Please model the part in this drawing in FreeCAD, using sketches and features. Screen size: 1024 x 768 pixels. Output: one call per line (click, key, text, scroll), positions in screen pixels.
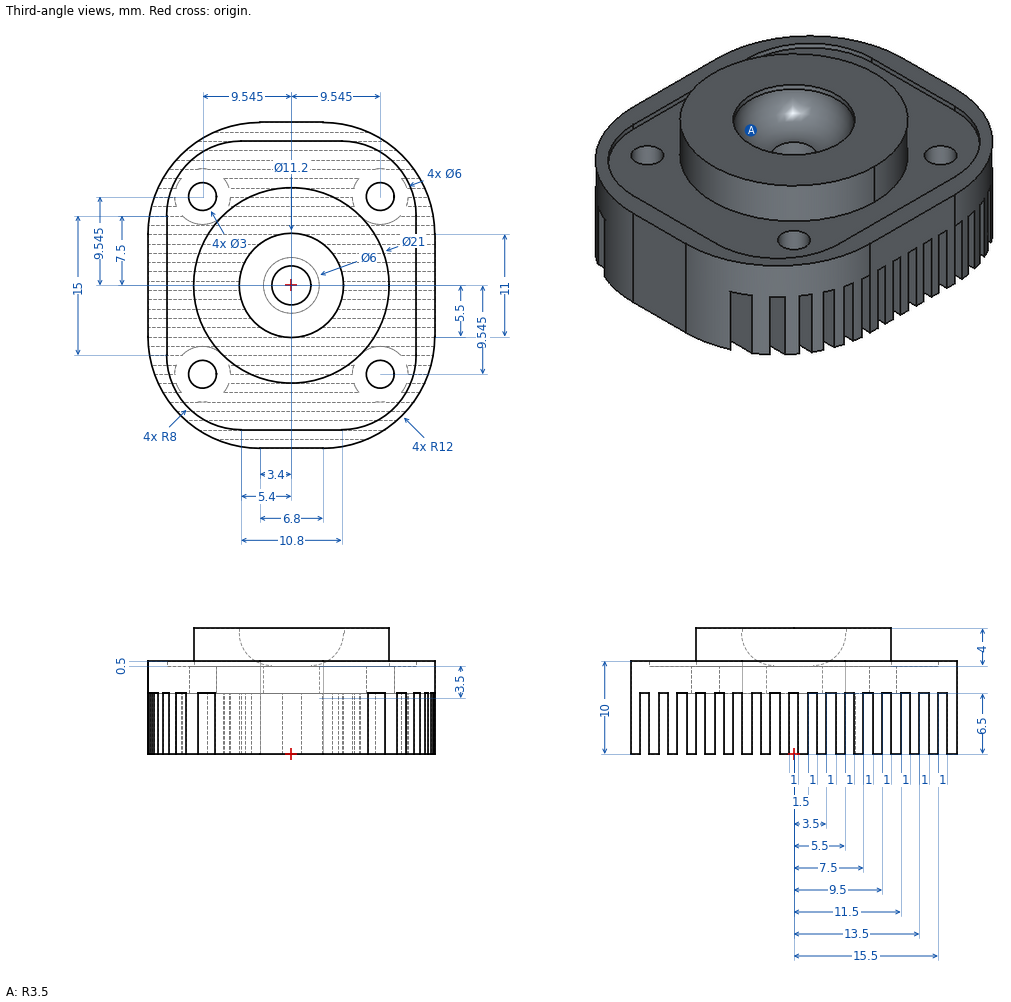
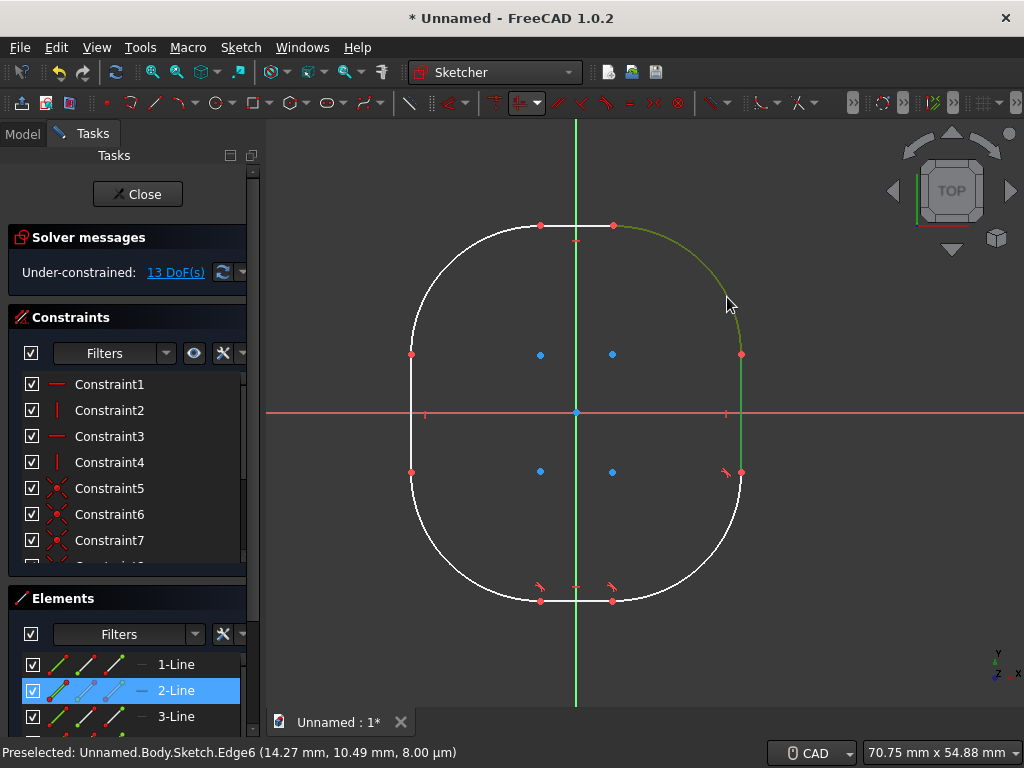
click(606, 104)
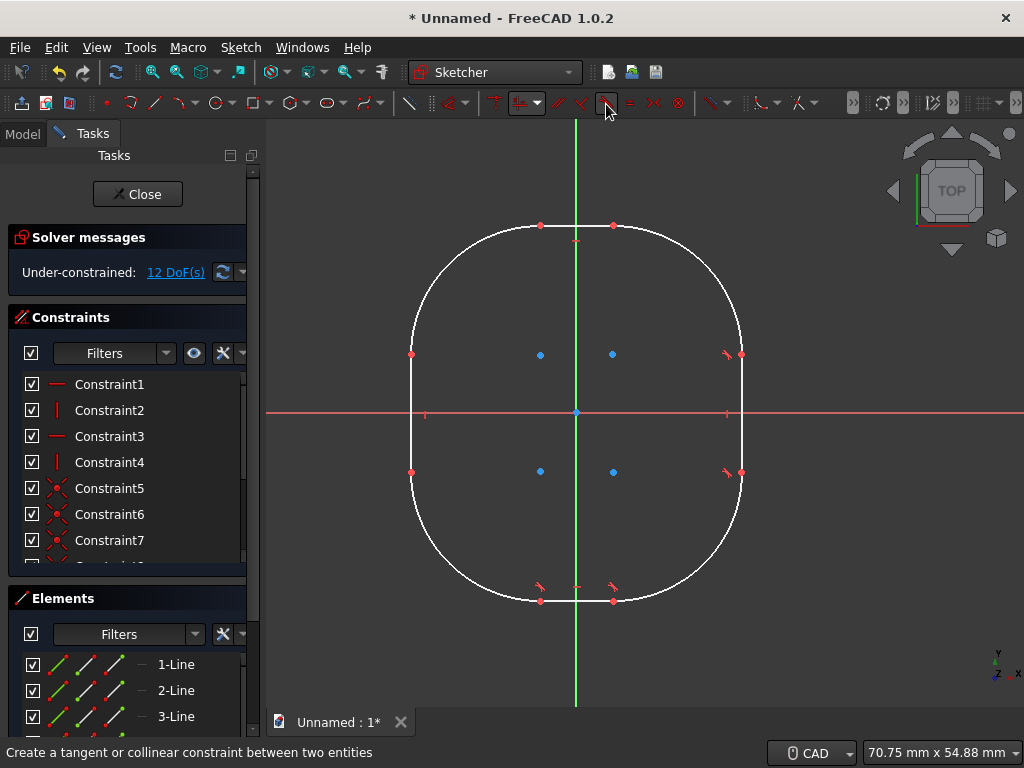
click(591, 226)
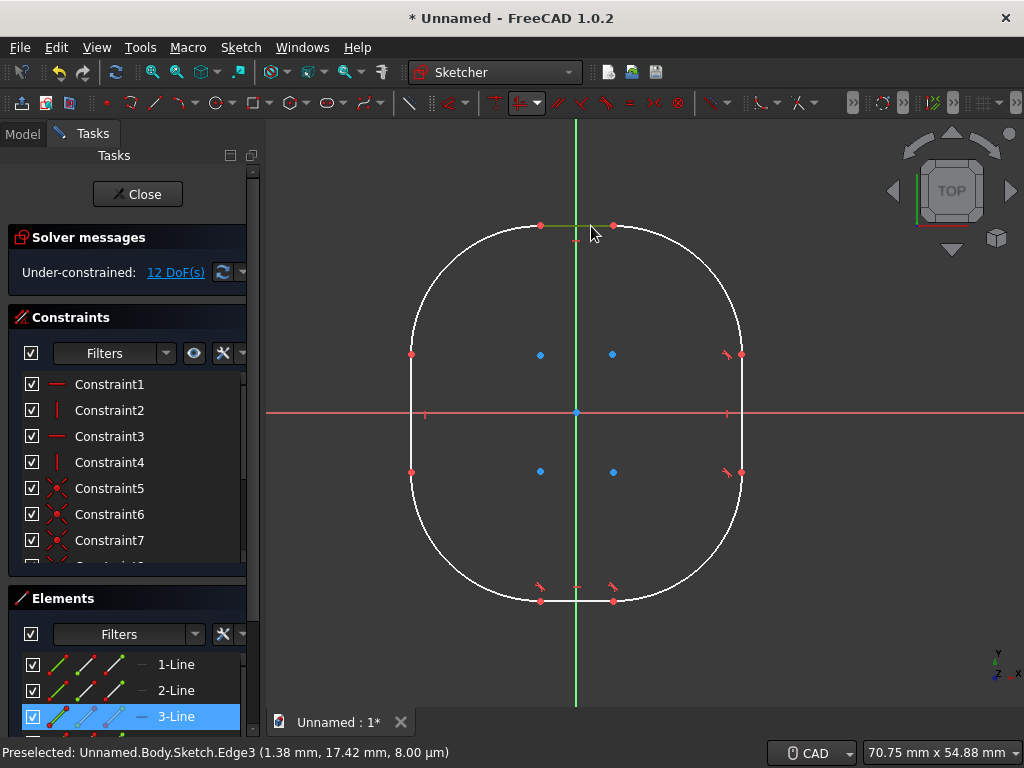
click(728, 296)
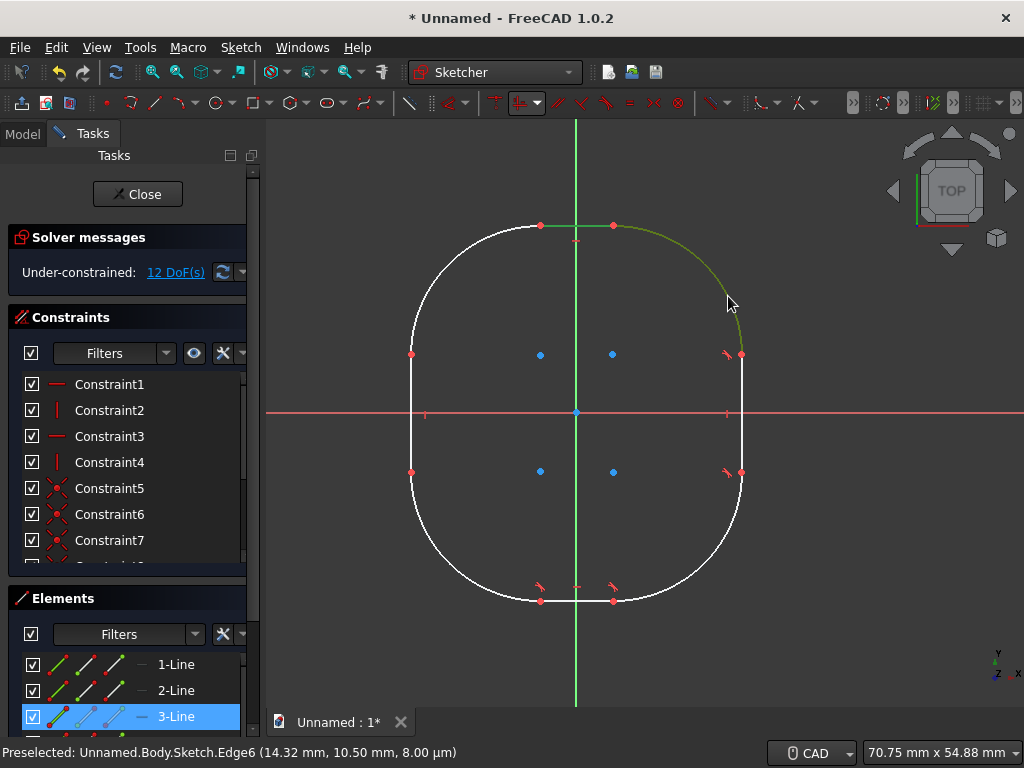
click(606, 104)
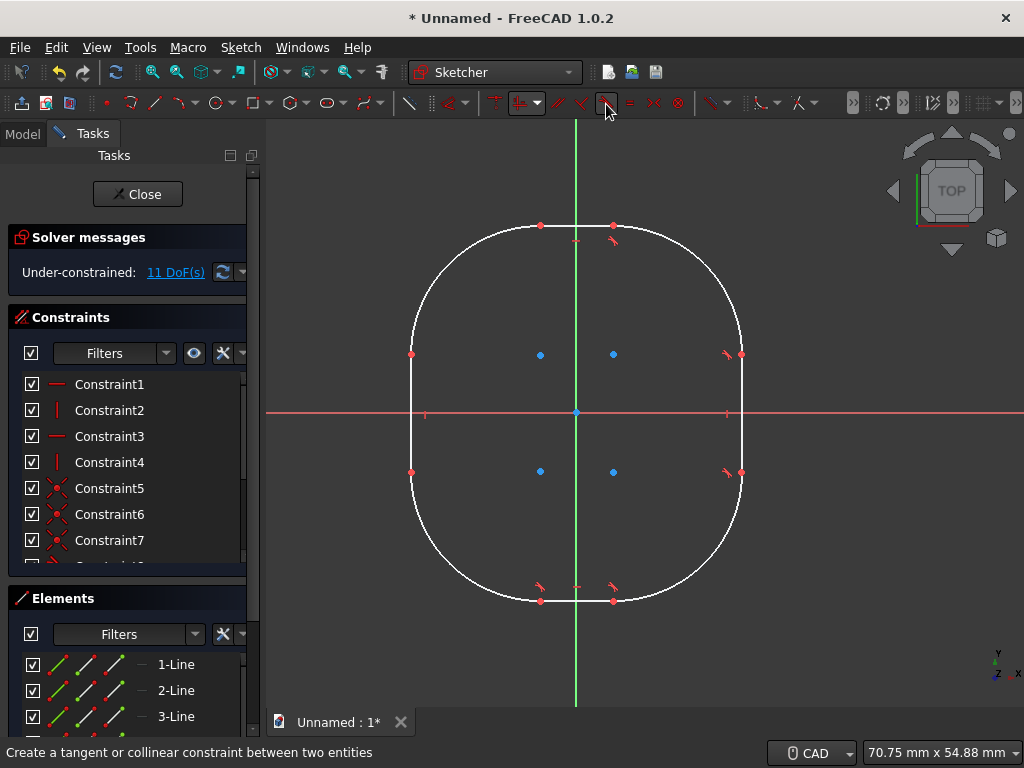
click(591, 226)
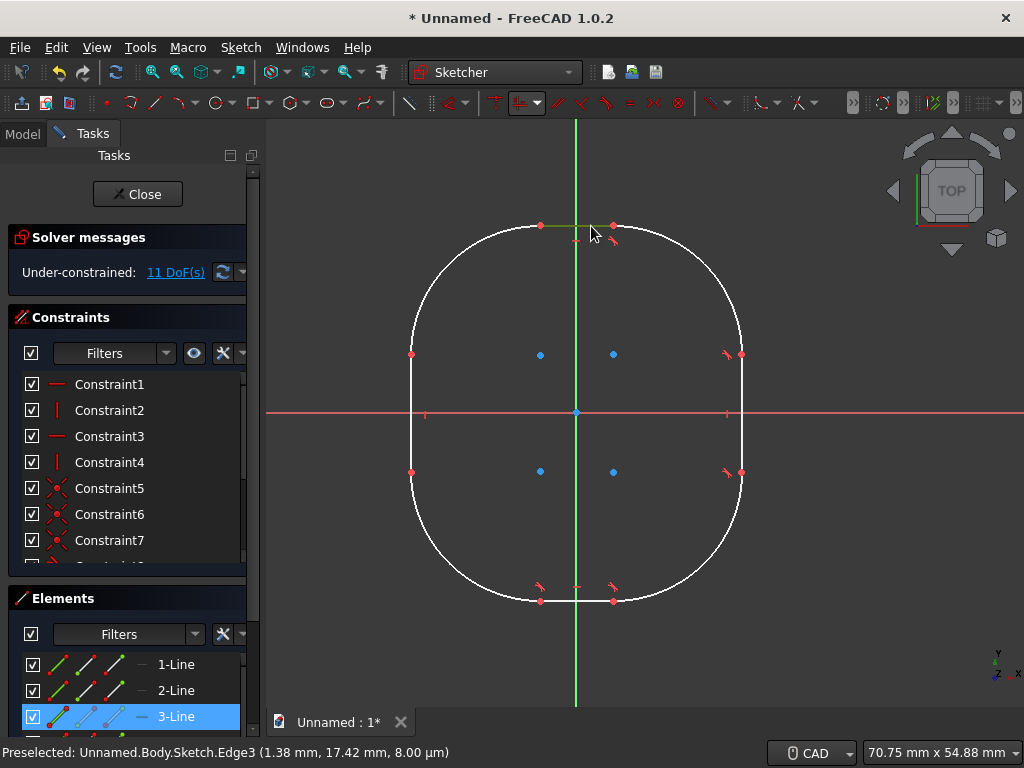
click(482, 240)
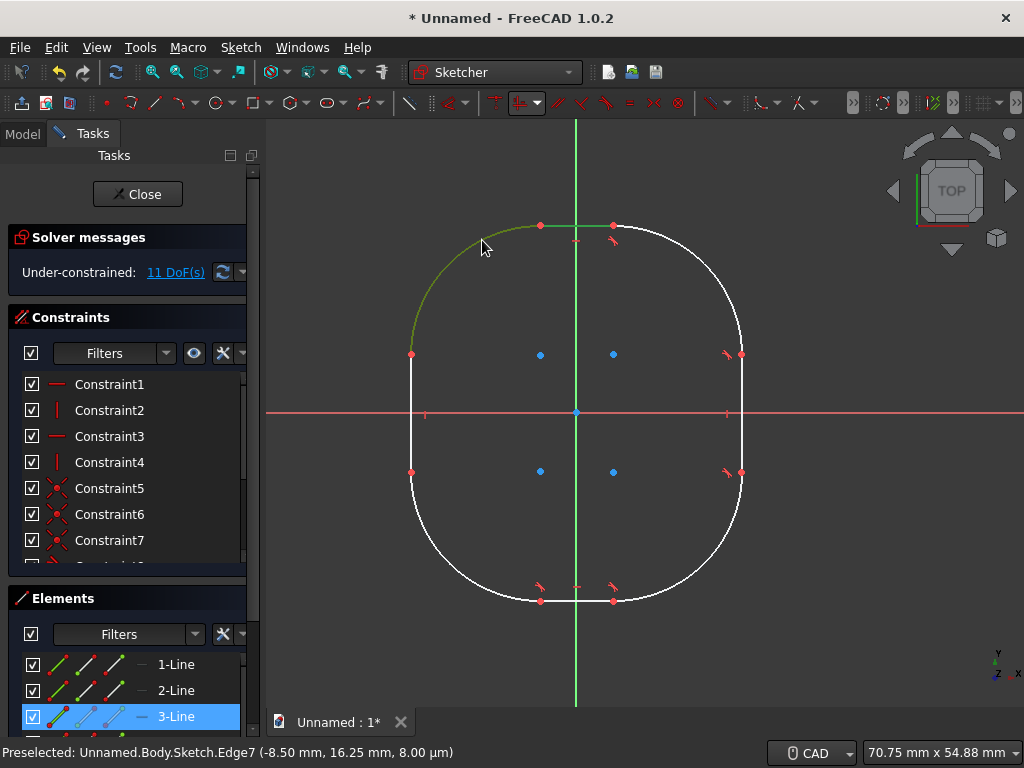
key(t)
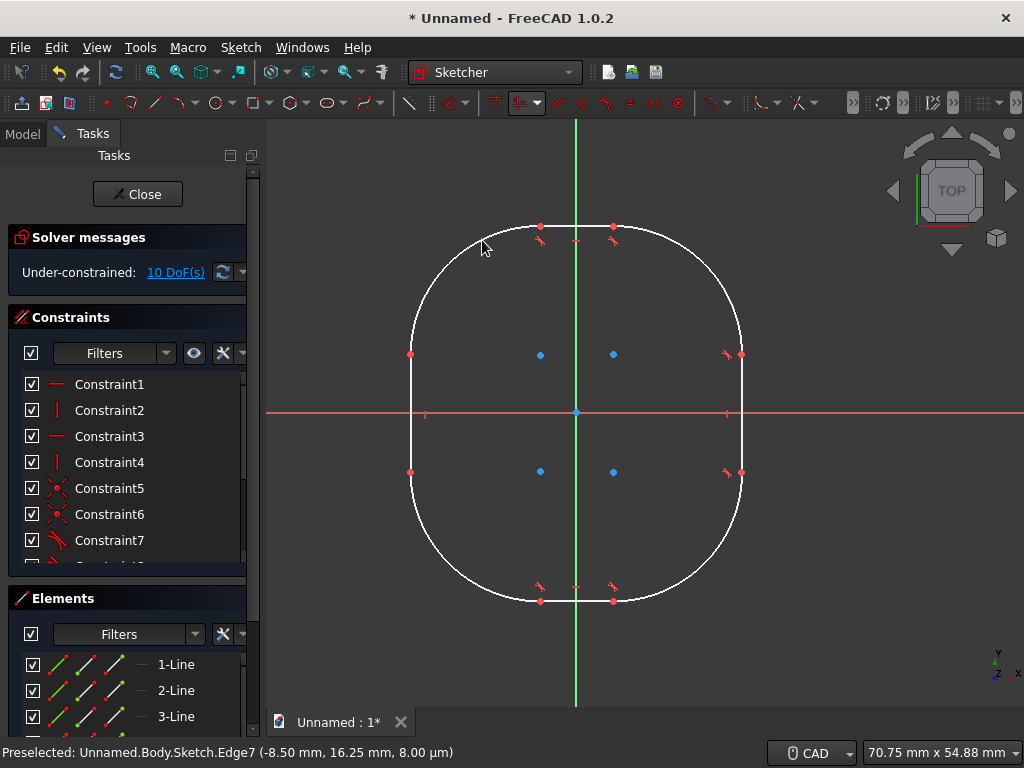
click(411, 390)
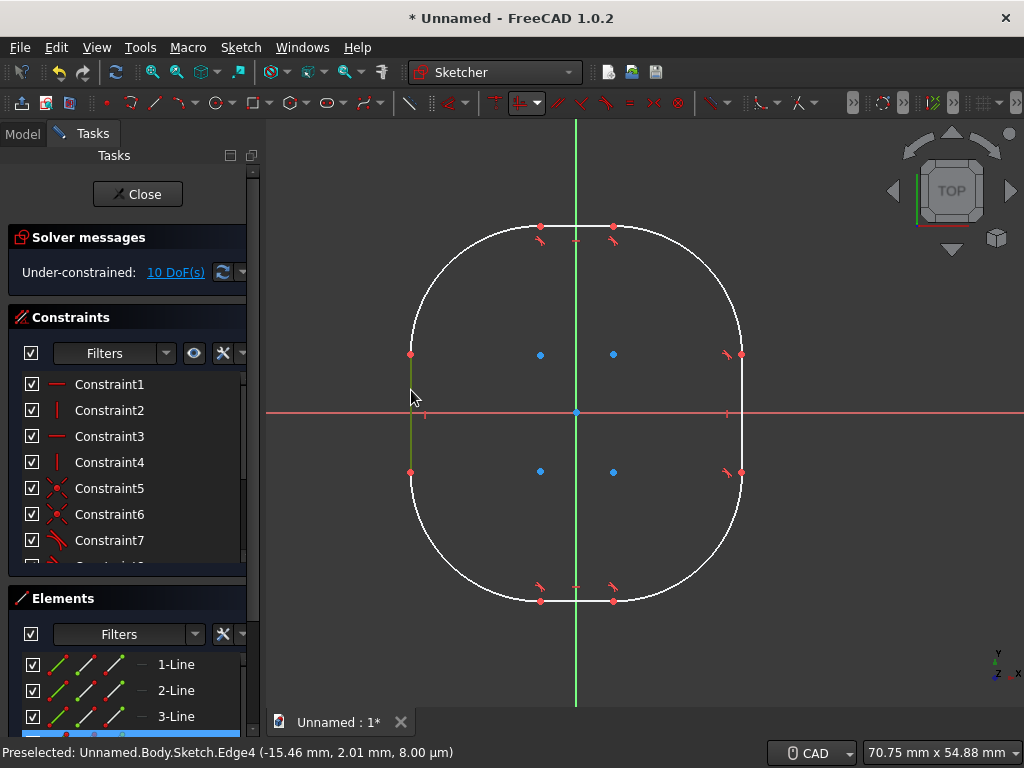
click(482, 240)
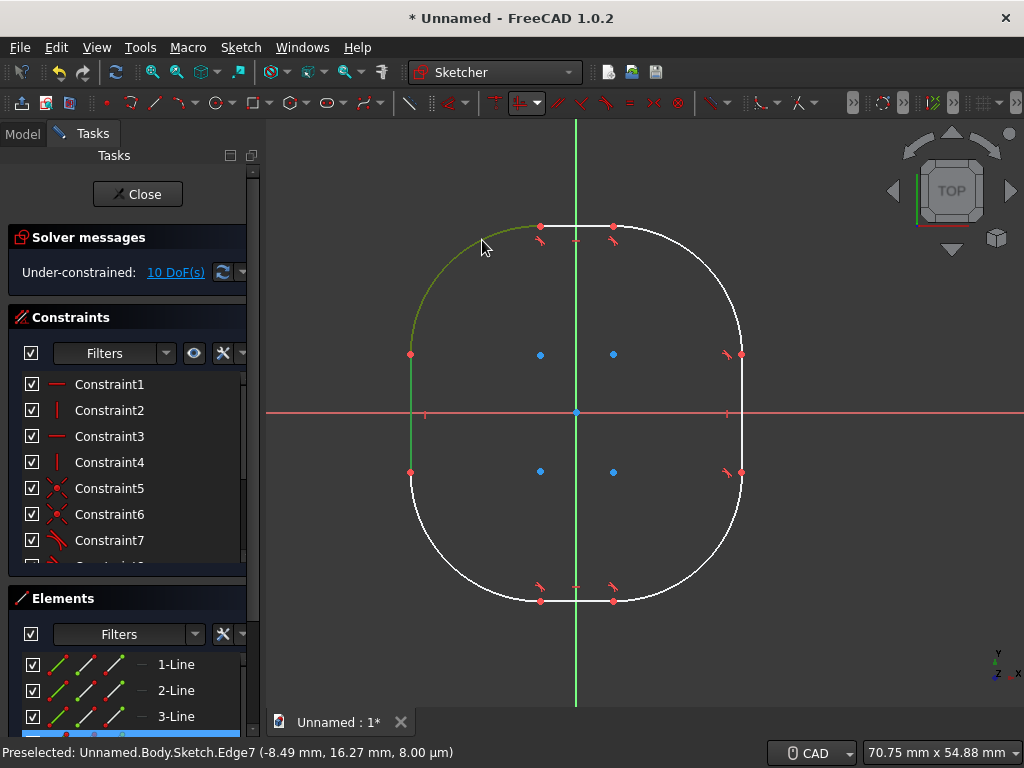
click(606, 104)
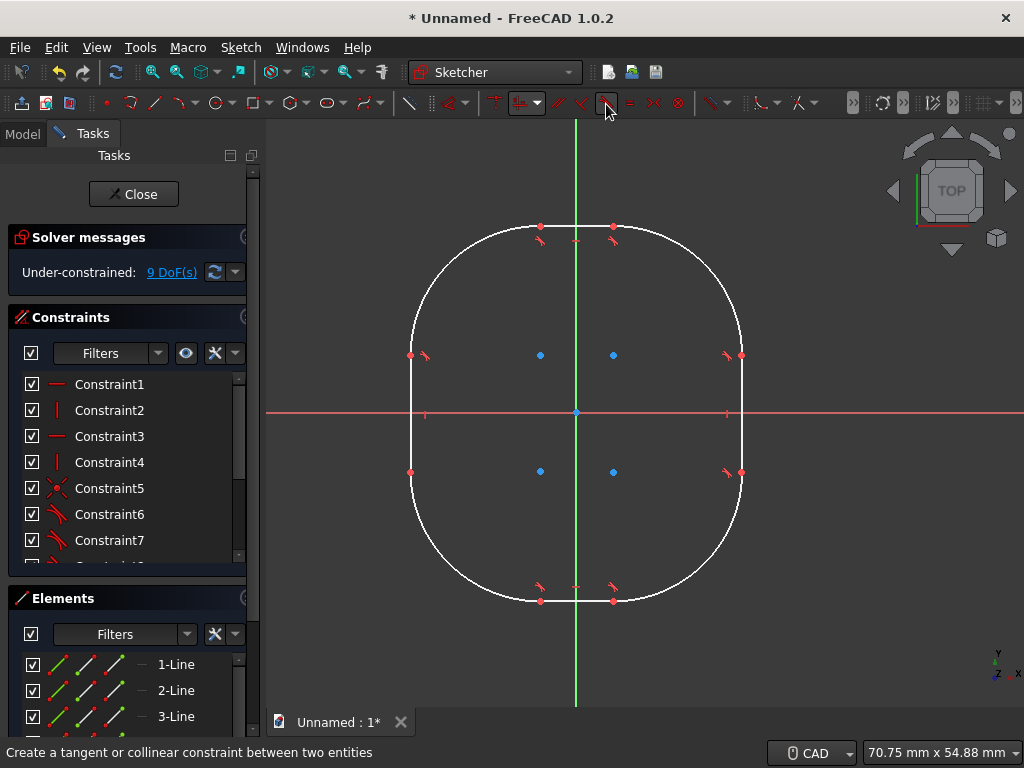
click(411, 391)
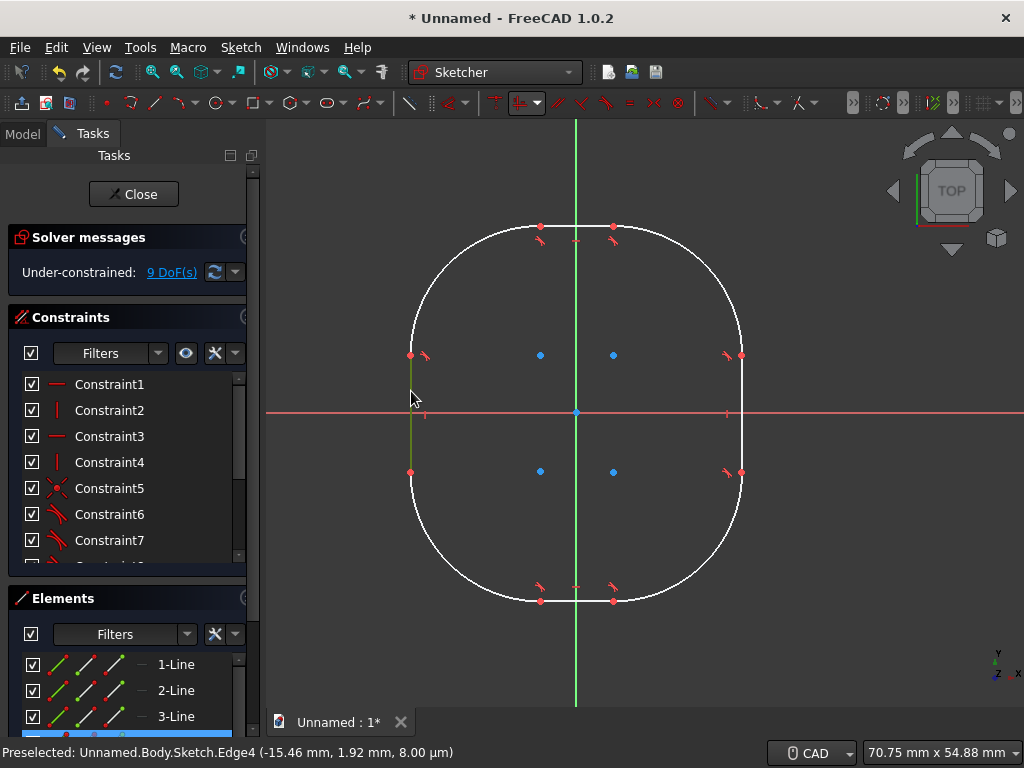
click(425, 531)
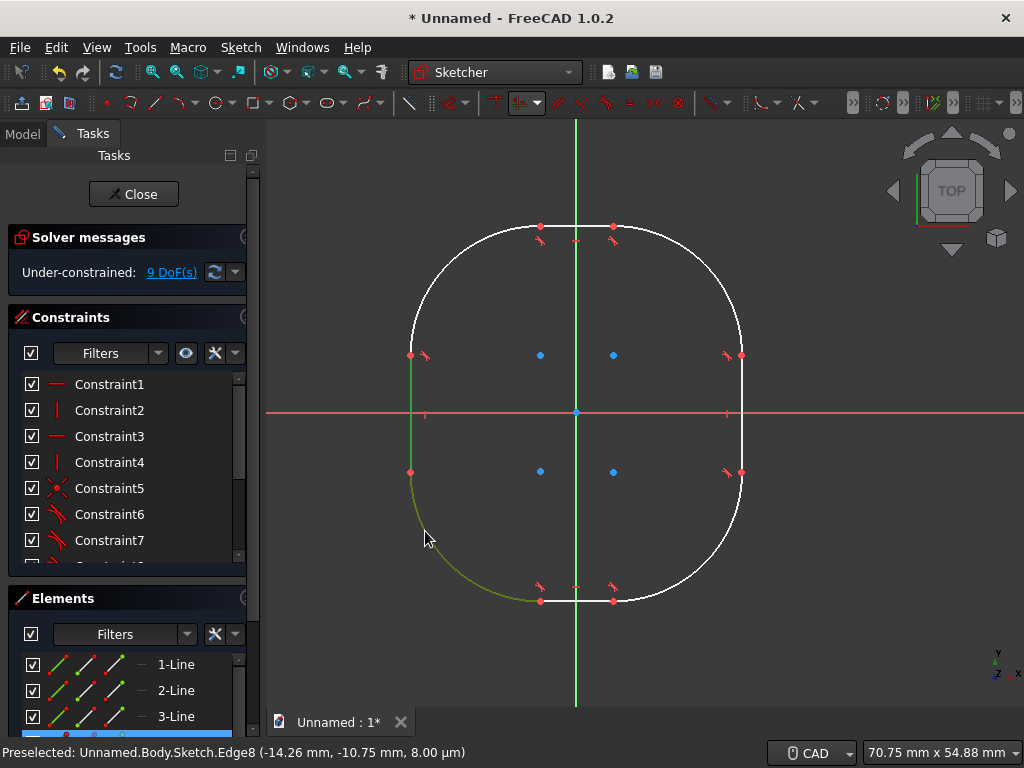
click(606, 104)